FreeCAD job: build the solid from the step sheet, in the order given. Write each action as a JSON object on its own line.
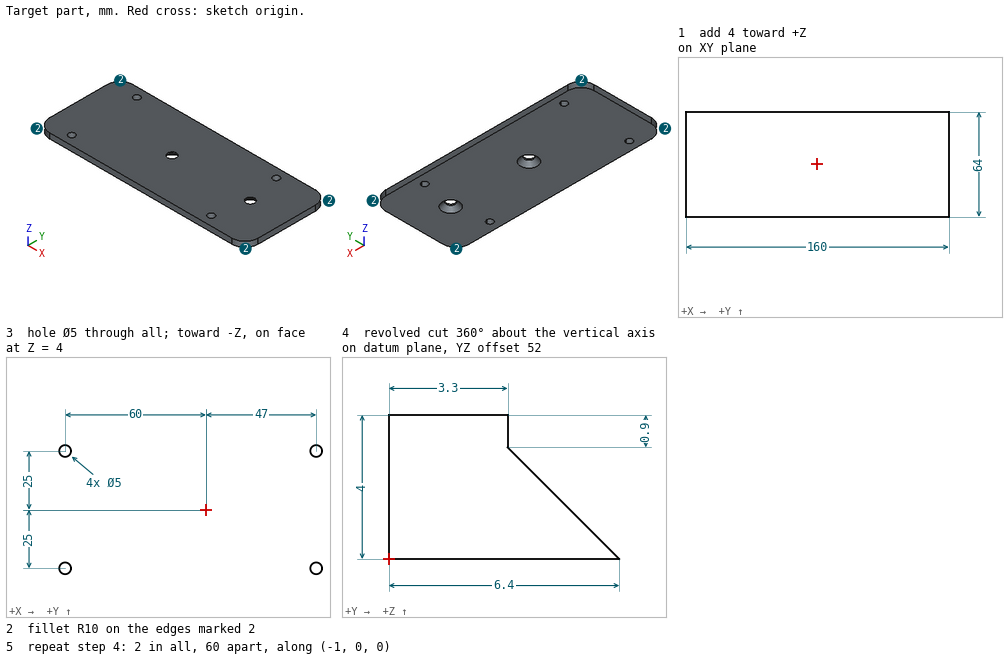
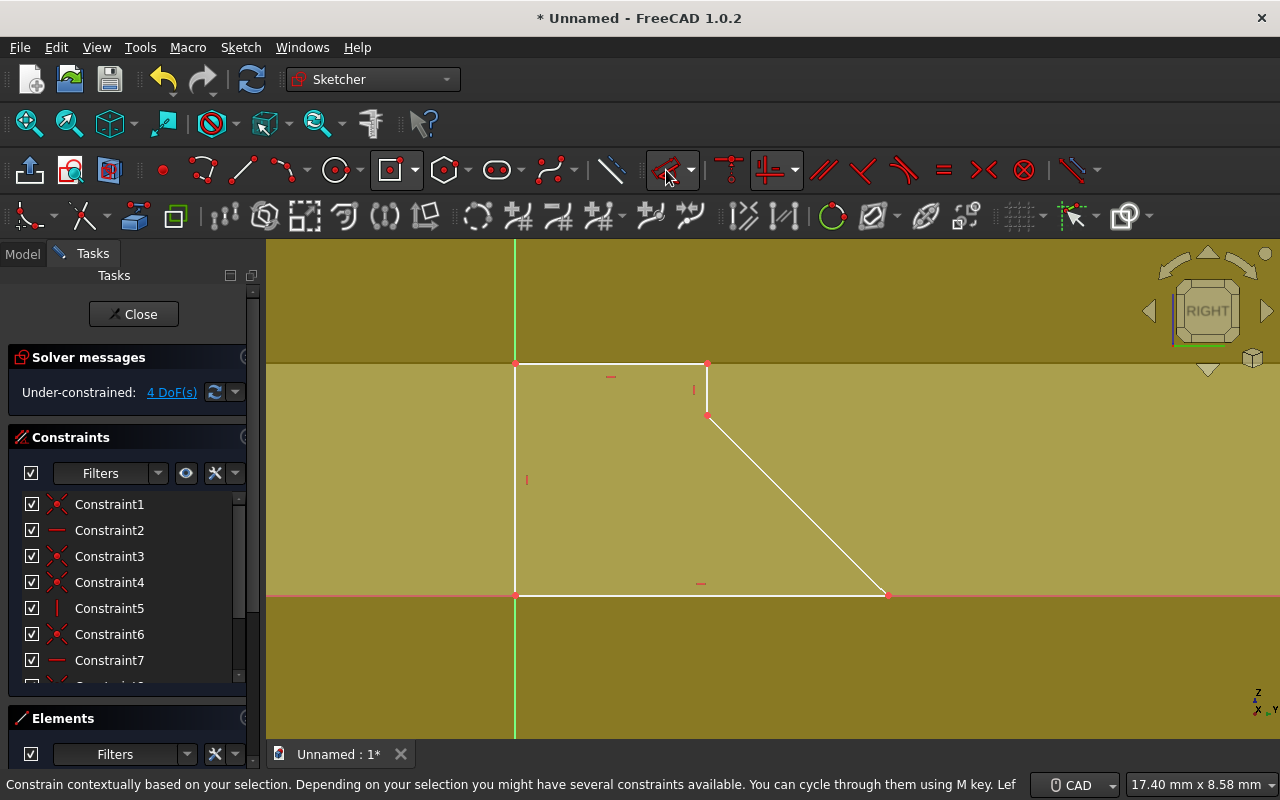
{"action": "left_click", "coordinate": [515, 434]}
{"action": "left_click", "coordinate": [481, 480]}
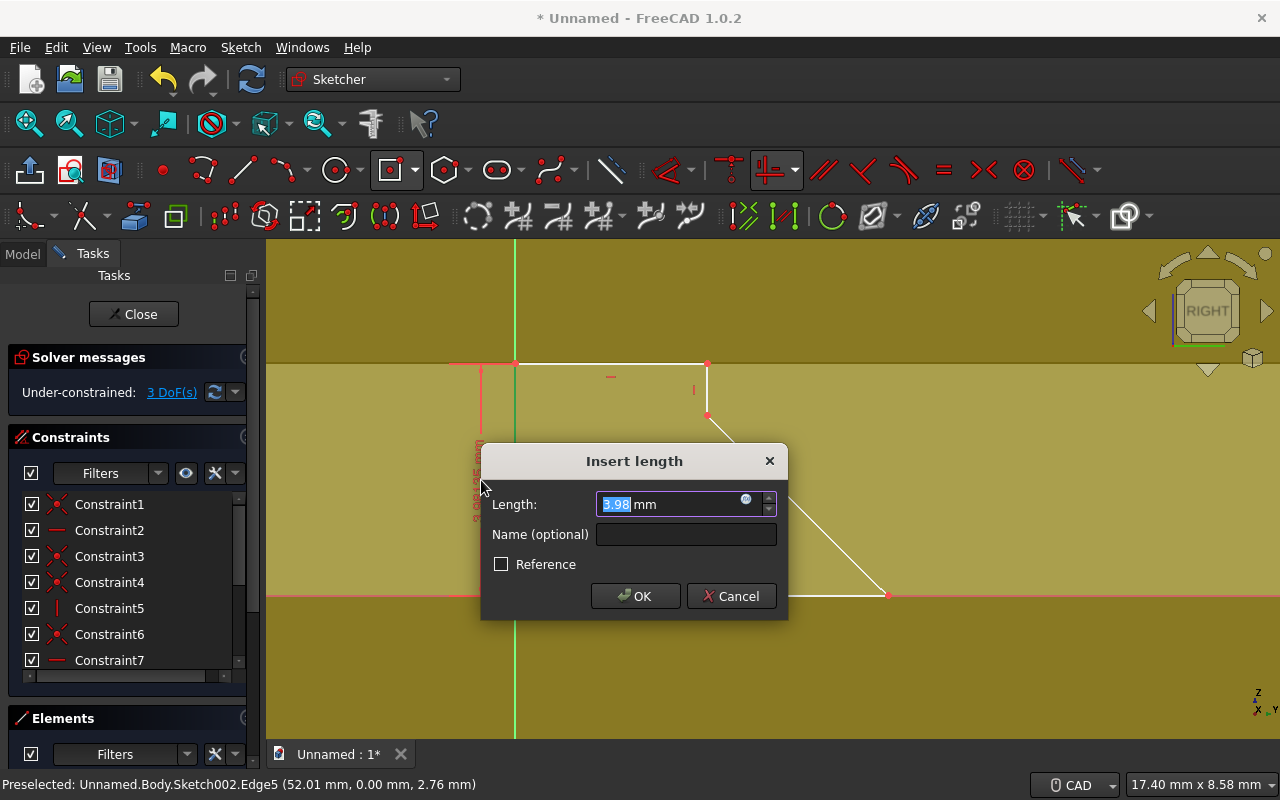
{"action": "type", "text": "4"}
{"action": "key", "text": "Return"}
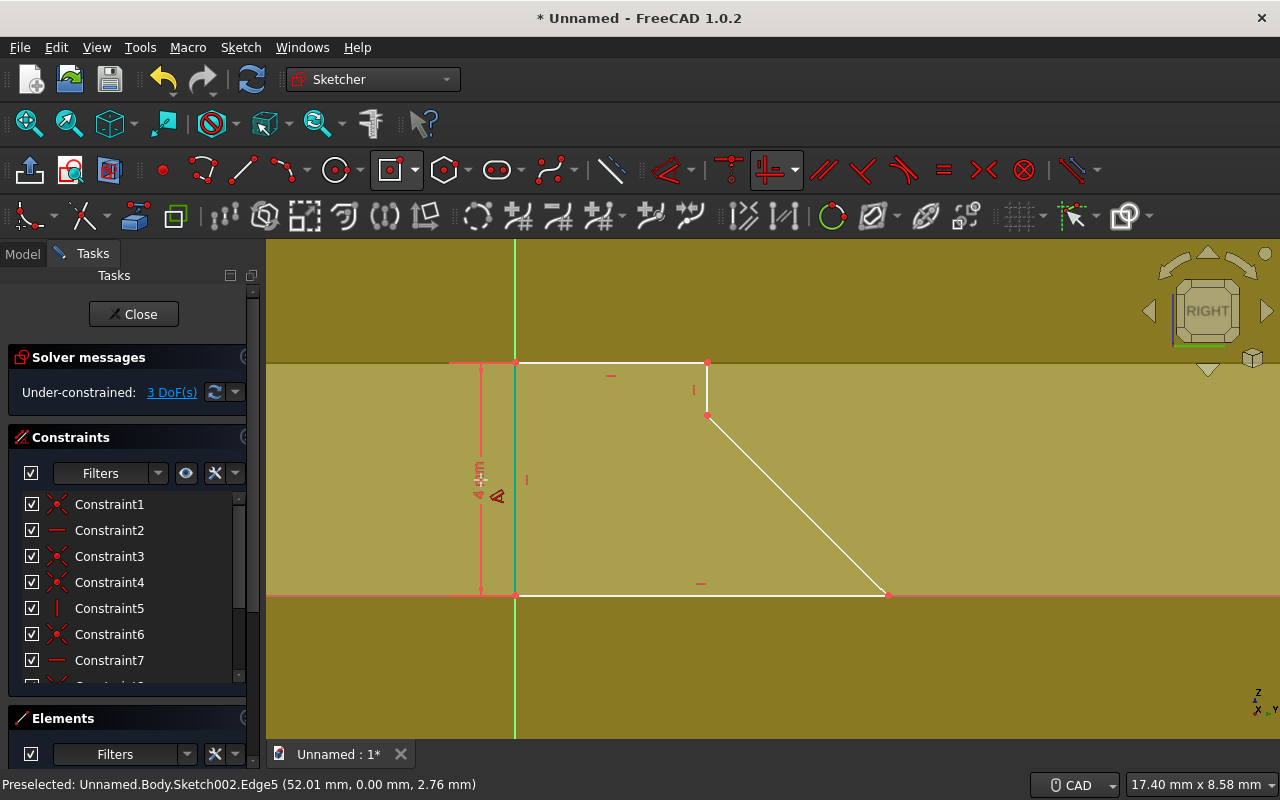
{"action": "left_click", "coordinate": [627, 596]}
{"action": "left_click", "coordinate": [702, 630]}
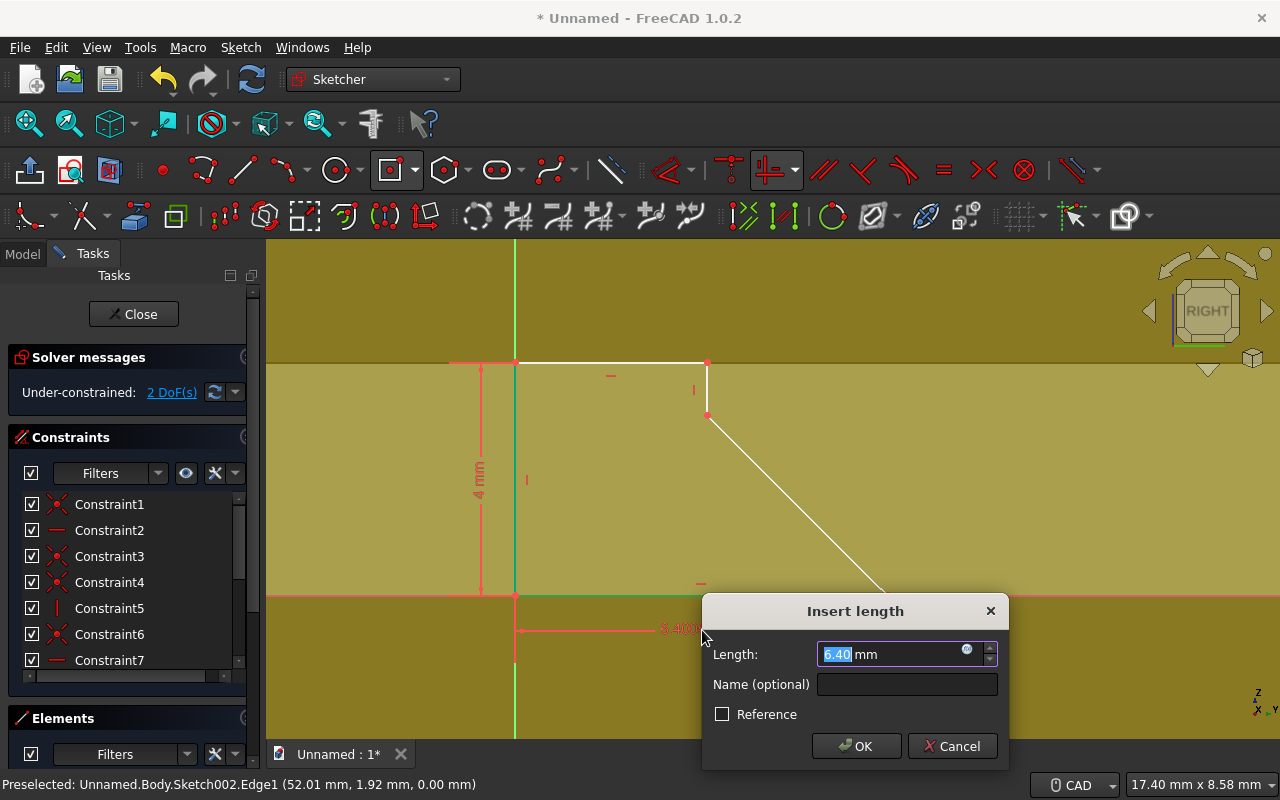
{"action": "type", "text": "6.4"}
{"action": "key", "text": "Return"}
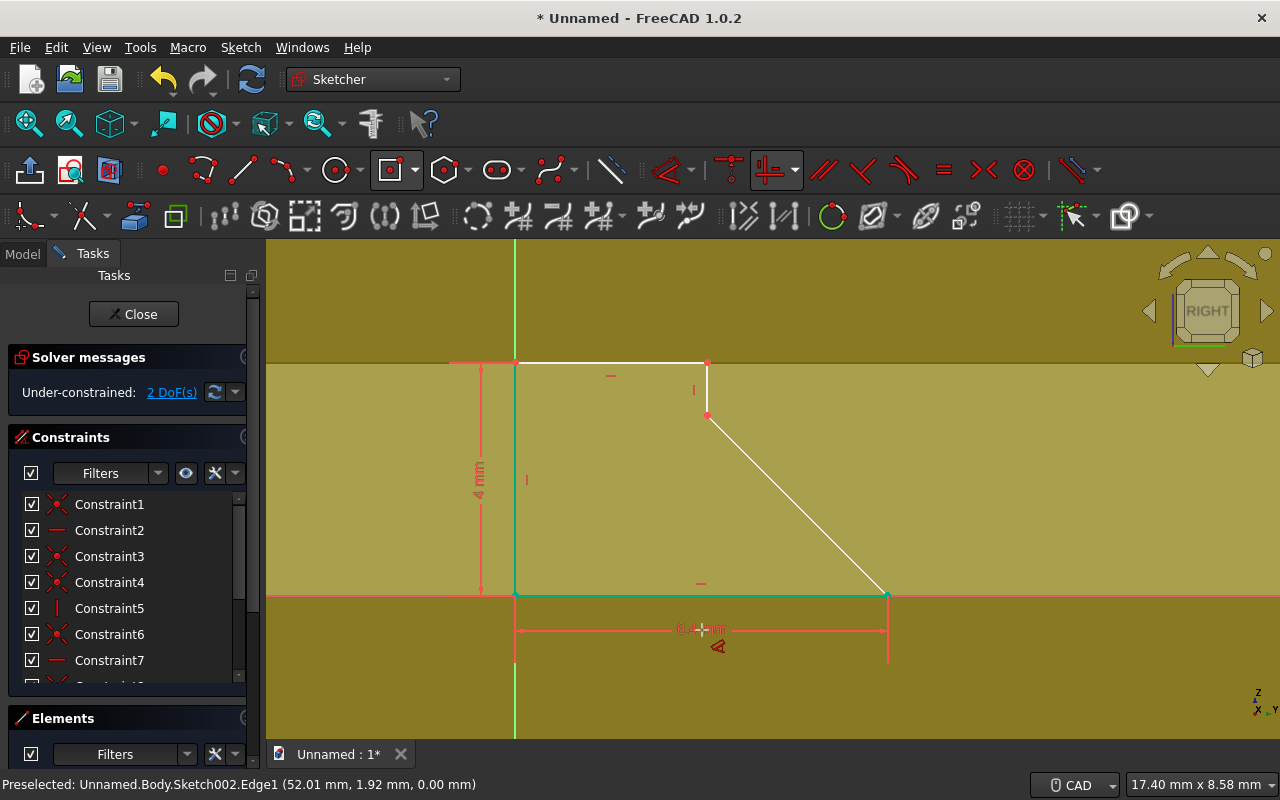
{"action": "left_click", "coordinate": [707, 400]}
{"action": "left_click", "coordinate": [741, 389]}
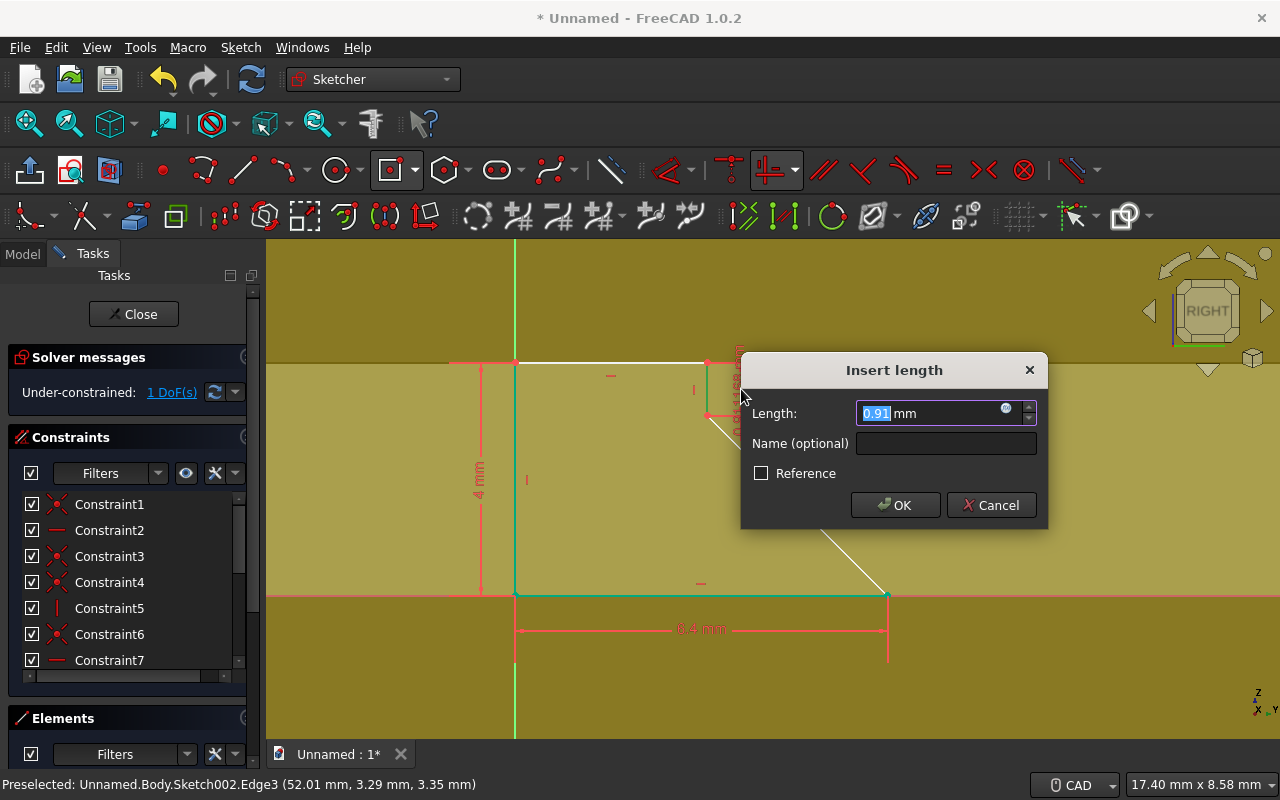
{"action": "type", "text": "0.9"}
{"action": "key", "text": "Return"}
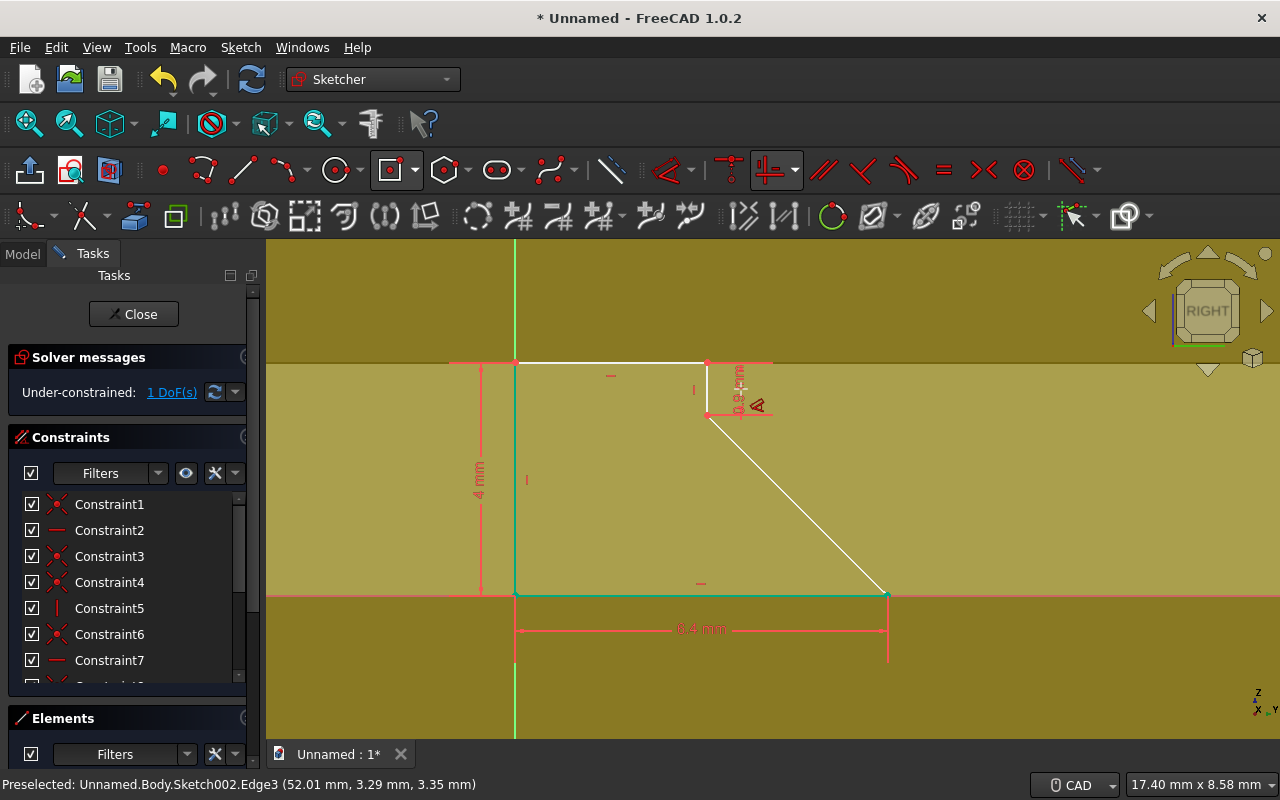
{"action": "left_click", "coordinate": [649, 363]}
{"action": "left_click", "coordinate": [611, 329]}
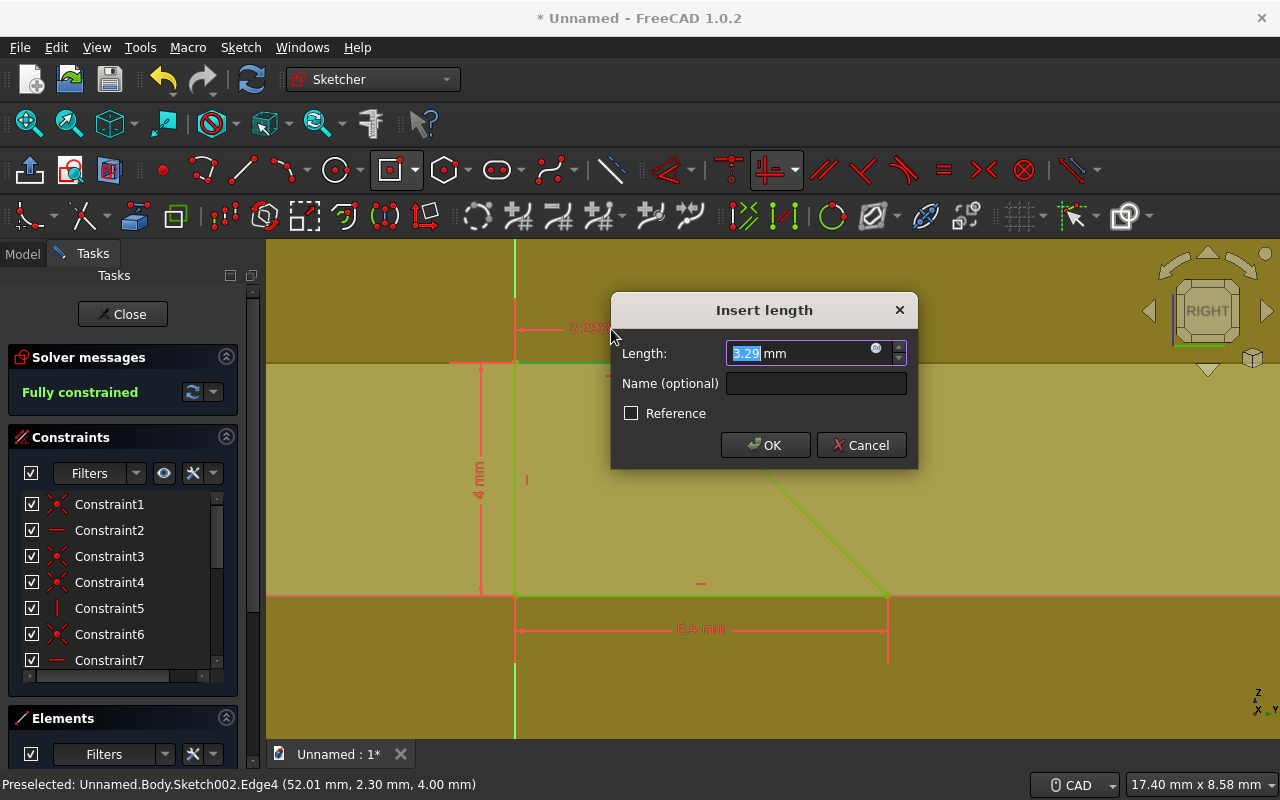
{"action": "type", "text": "3.3"}
{"action": "key", "text": "Return"}
{"action": "key", "text": "Escape"}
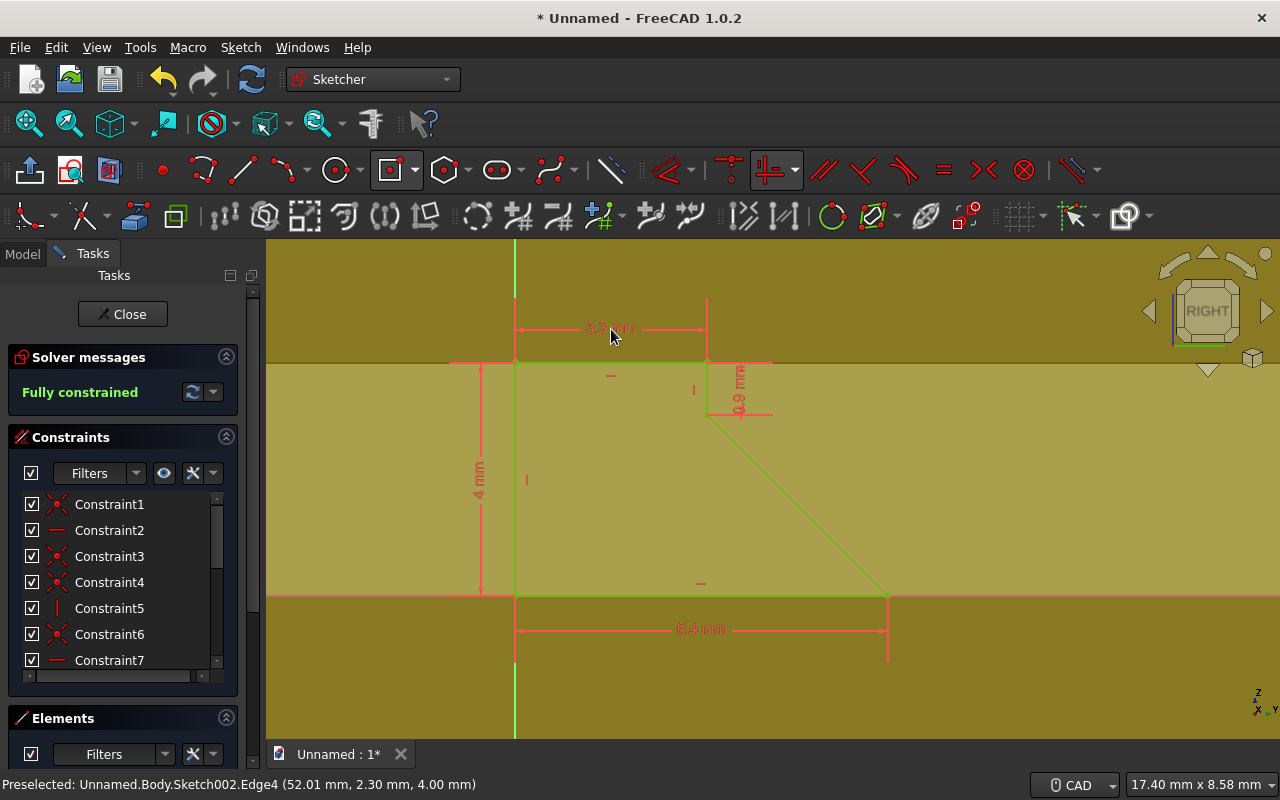
{"action": "left_click", "coordinate": [123, 314]}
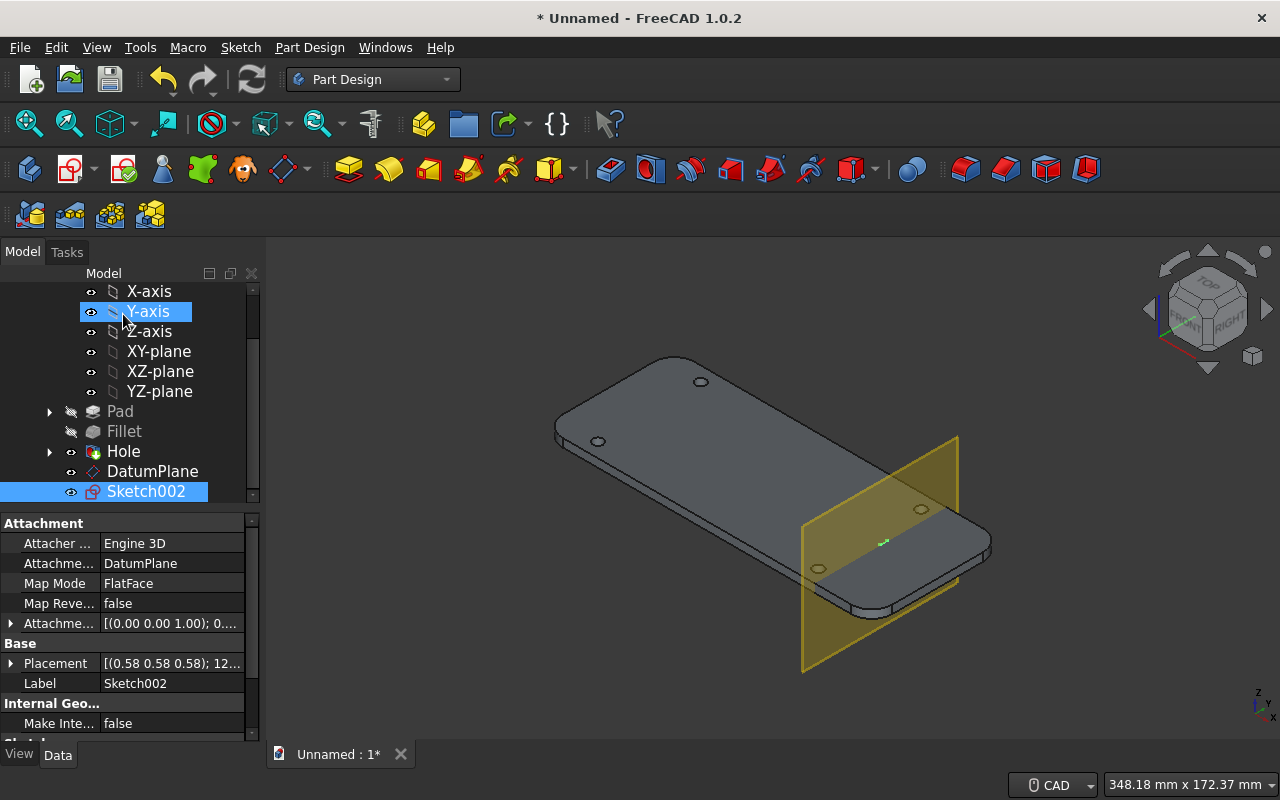
{"action": "left_click", "coordinate": [692, 170]}